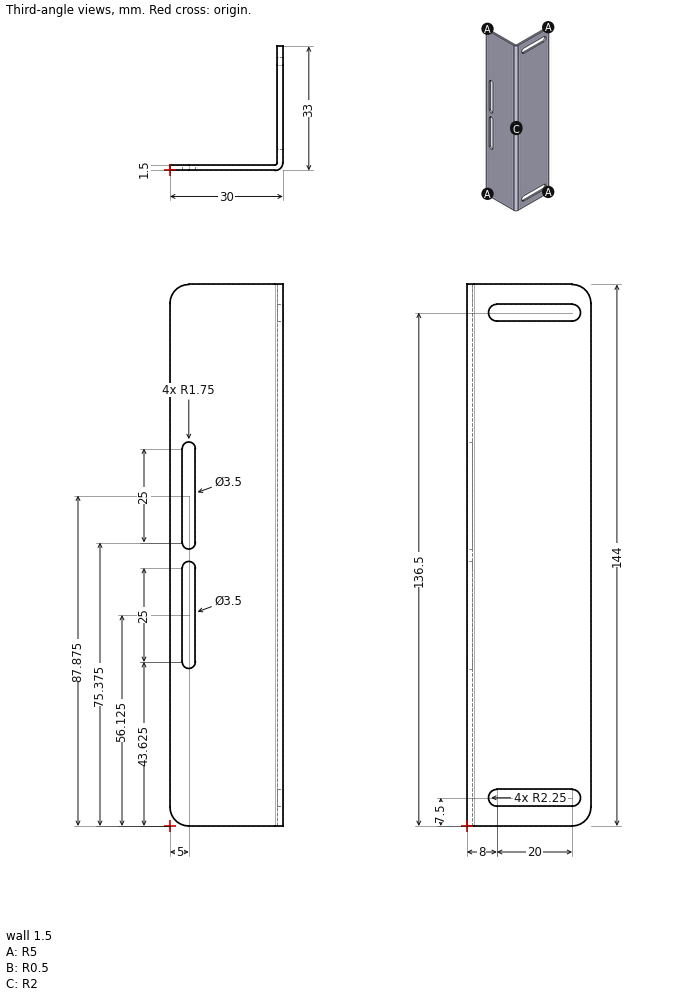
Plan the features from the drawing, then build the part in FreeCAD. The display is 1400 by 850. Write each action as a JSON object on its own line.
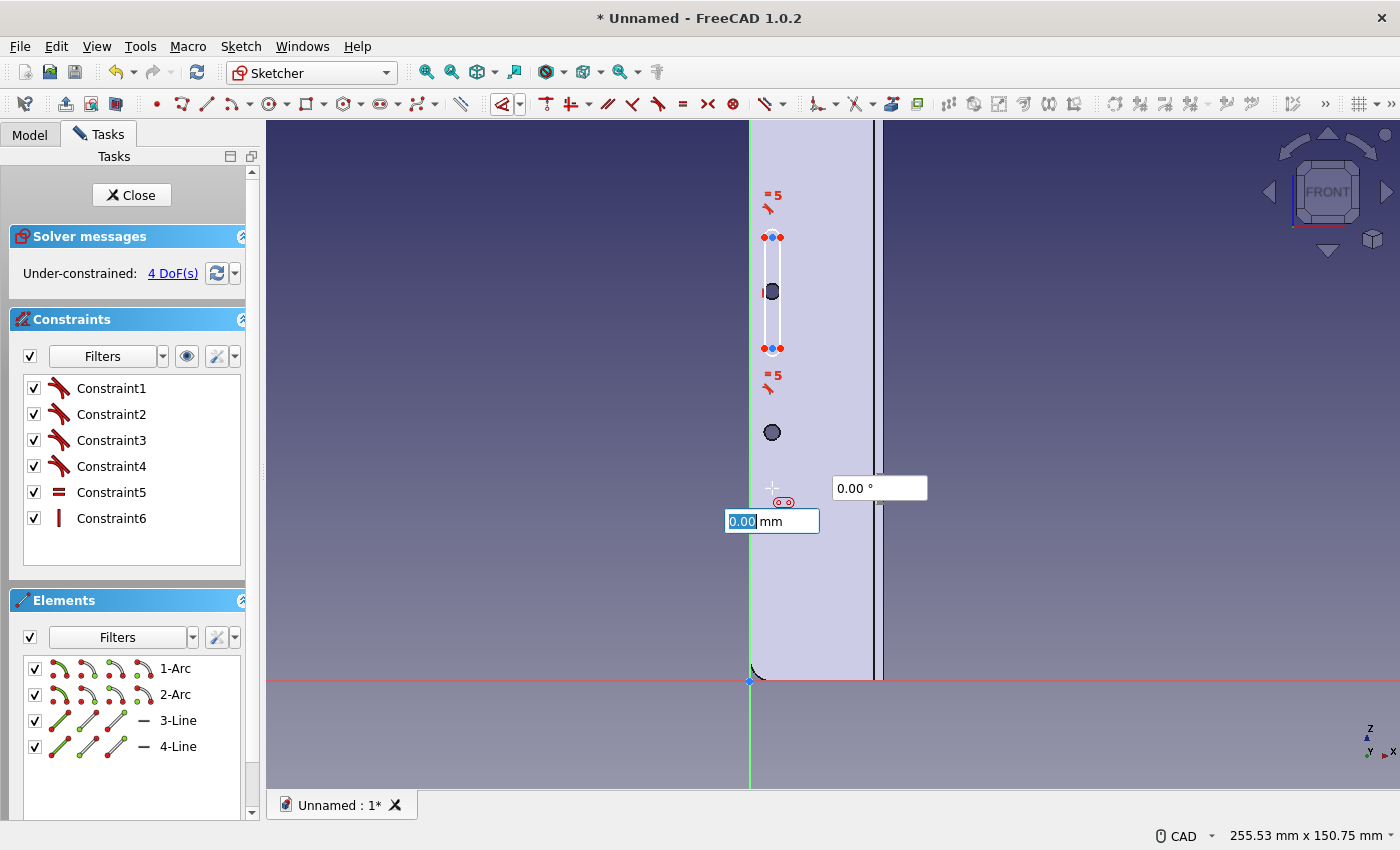
{"action": "left_click", "coordinate": [772, 377]}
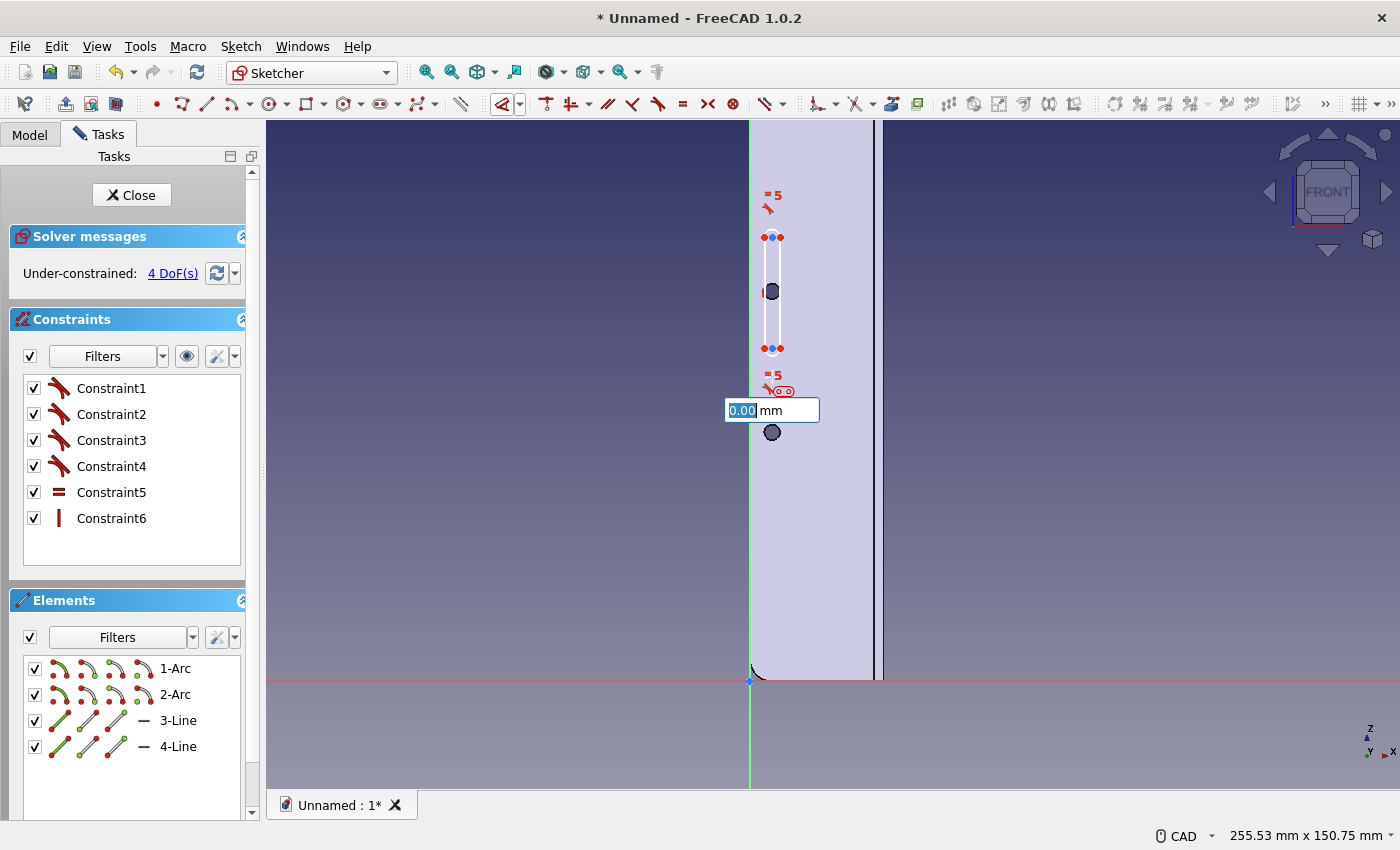
{"action": "scroll", "coordinate": [764, 432], "scroll_direction": "up", "scroll_amount": 4}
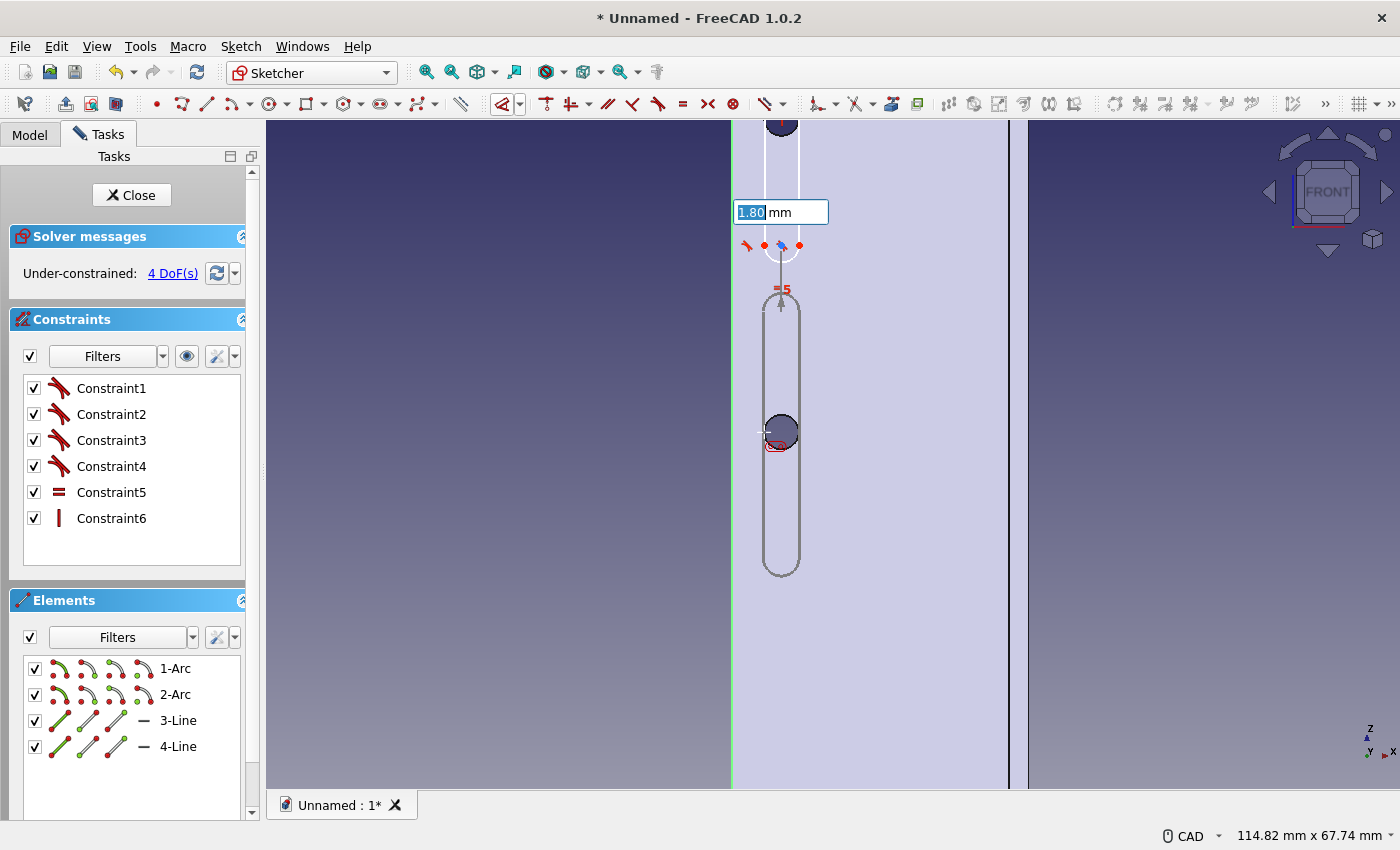
{"action": "left_click", "coordinate": [764, 432]}
{"action": "key", "text": "Escape"}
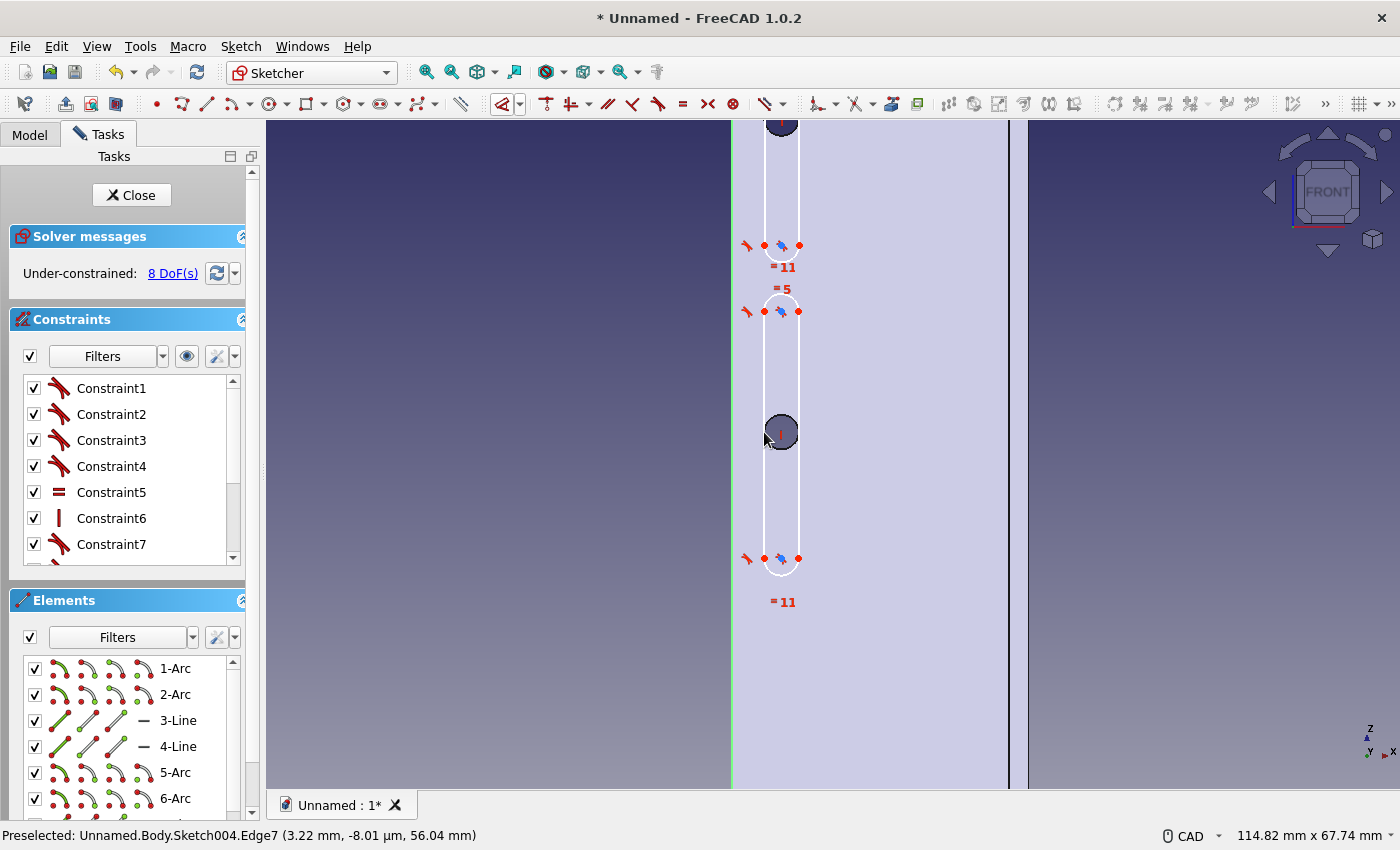
{"action": "left_click", "coordinate": [768, 255]}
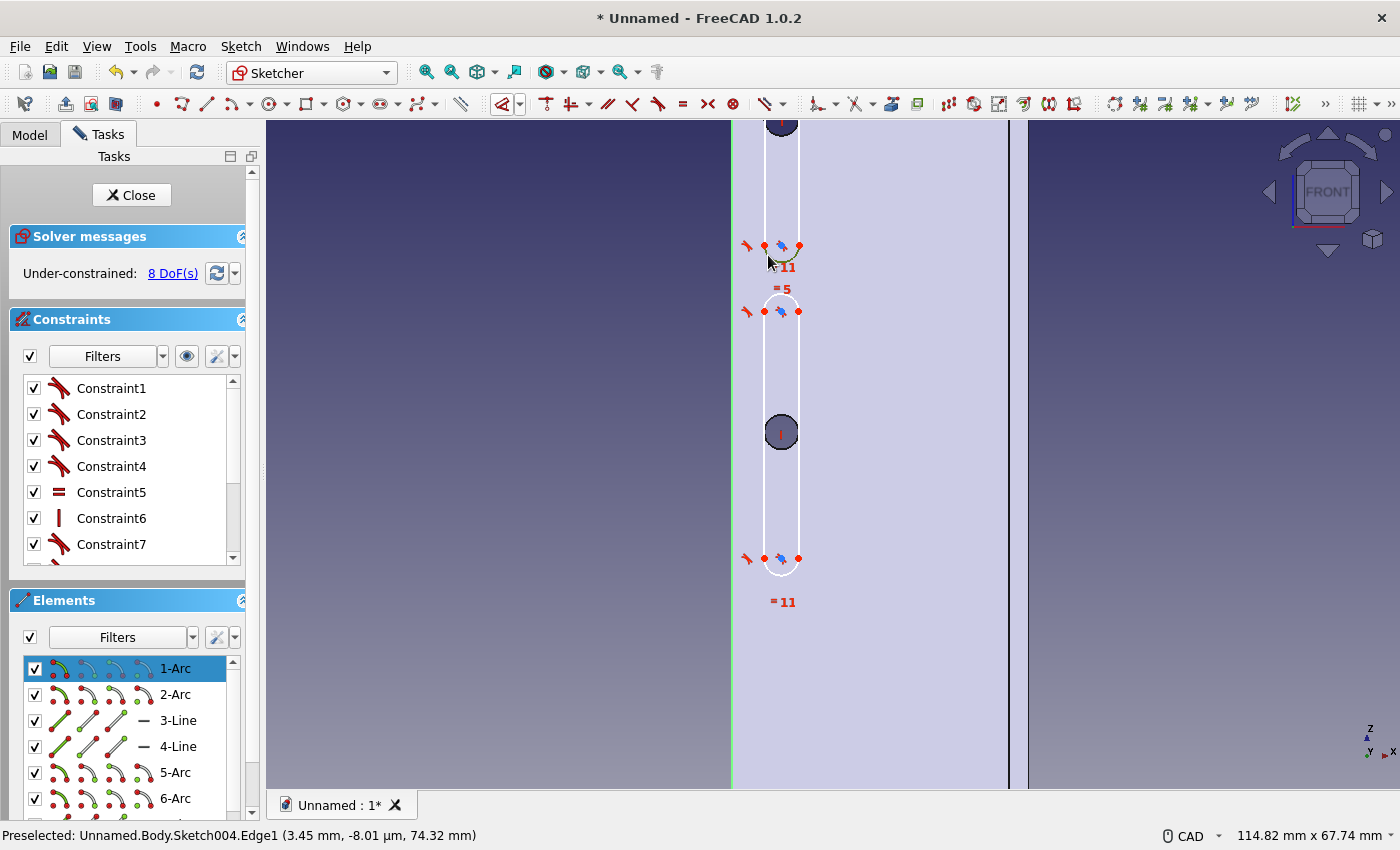
{"action": "left_click", "coordinate": [771, 572]}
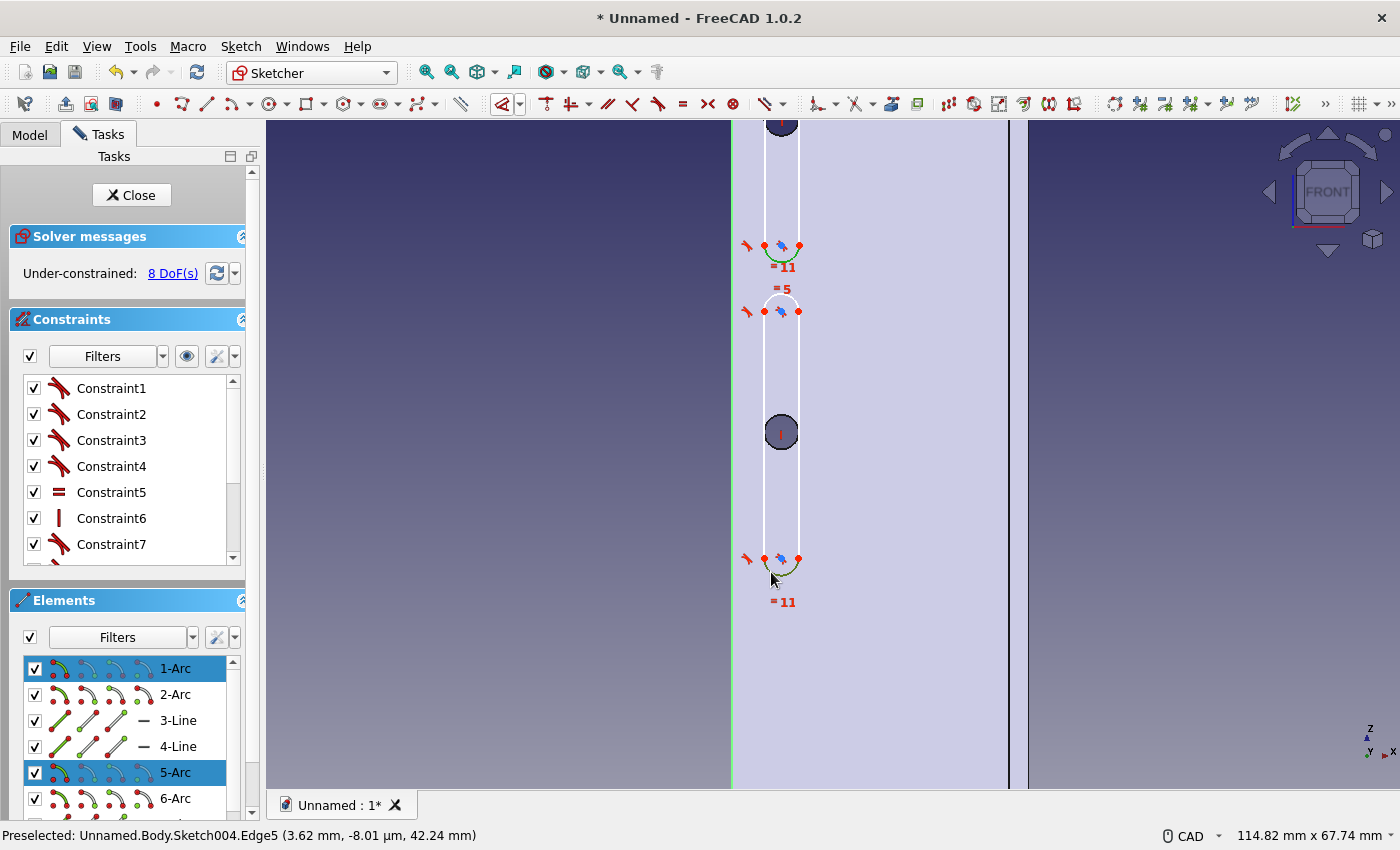
{"action": "left_click", "coordinate": [683, 104]}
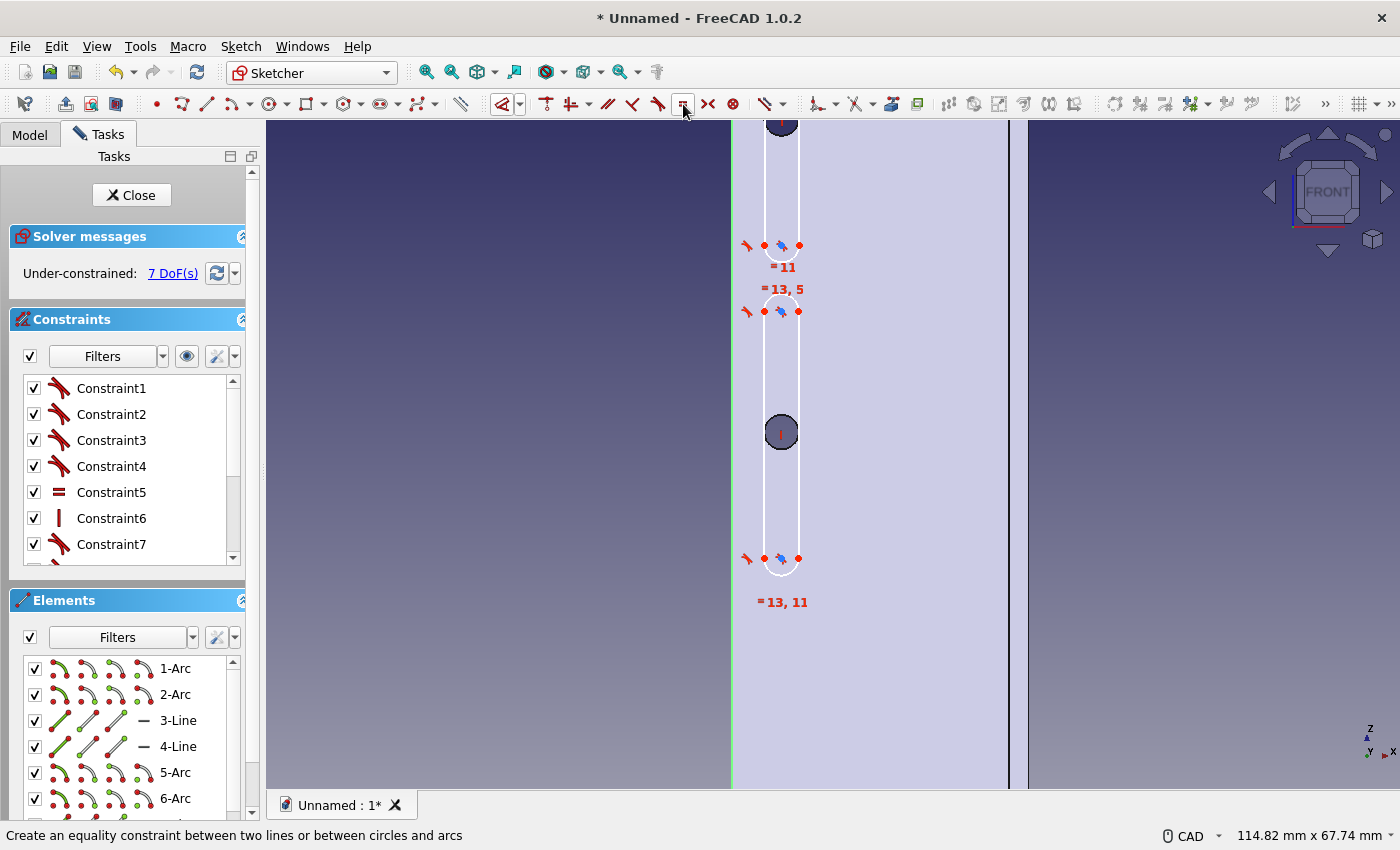
{"action": "scroll", "coordinate": [772, 259], "scroll_direction": "up", "scroll_amount": 5}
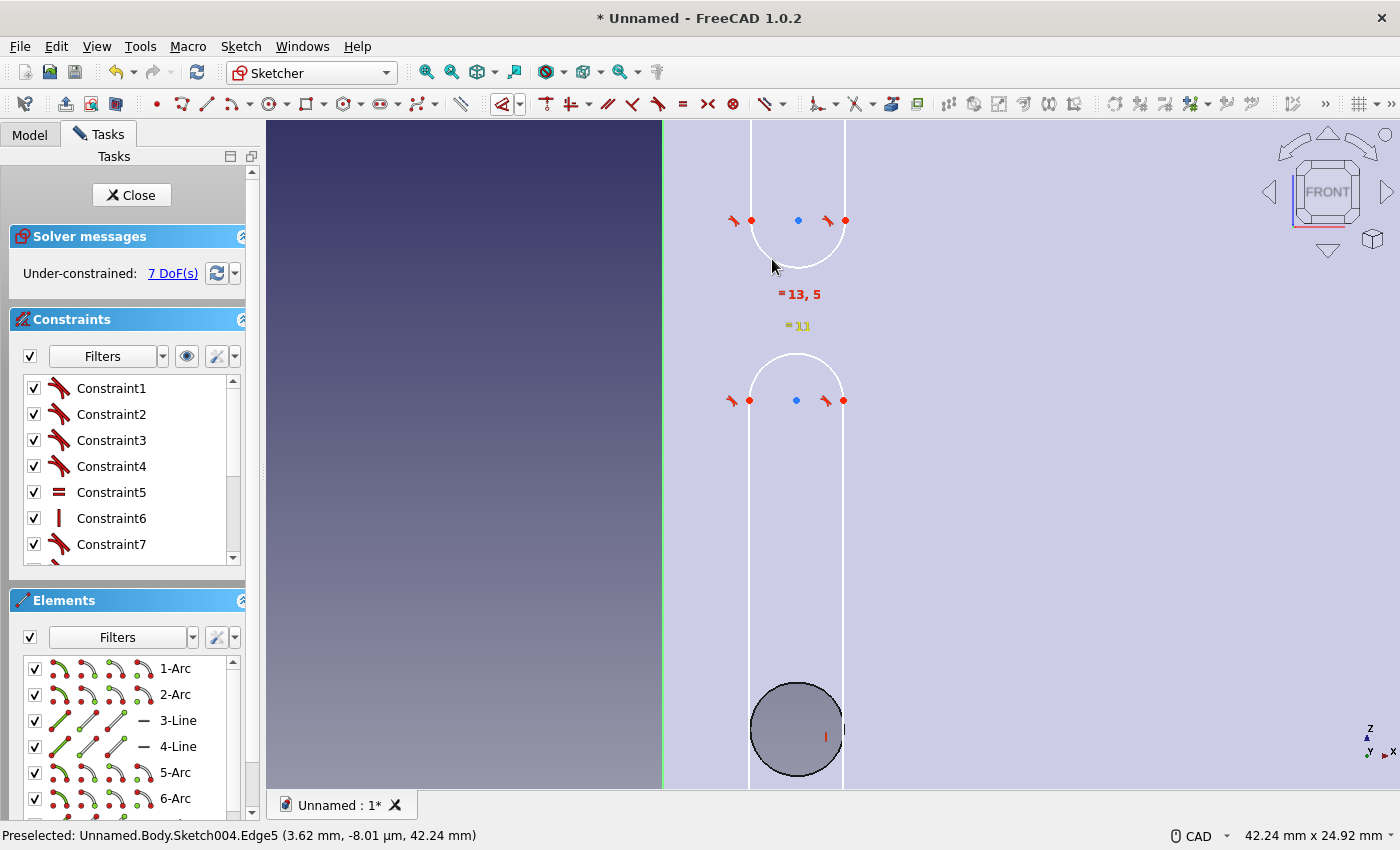
{"action": "left_click", "coordinate": [771, 259]}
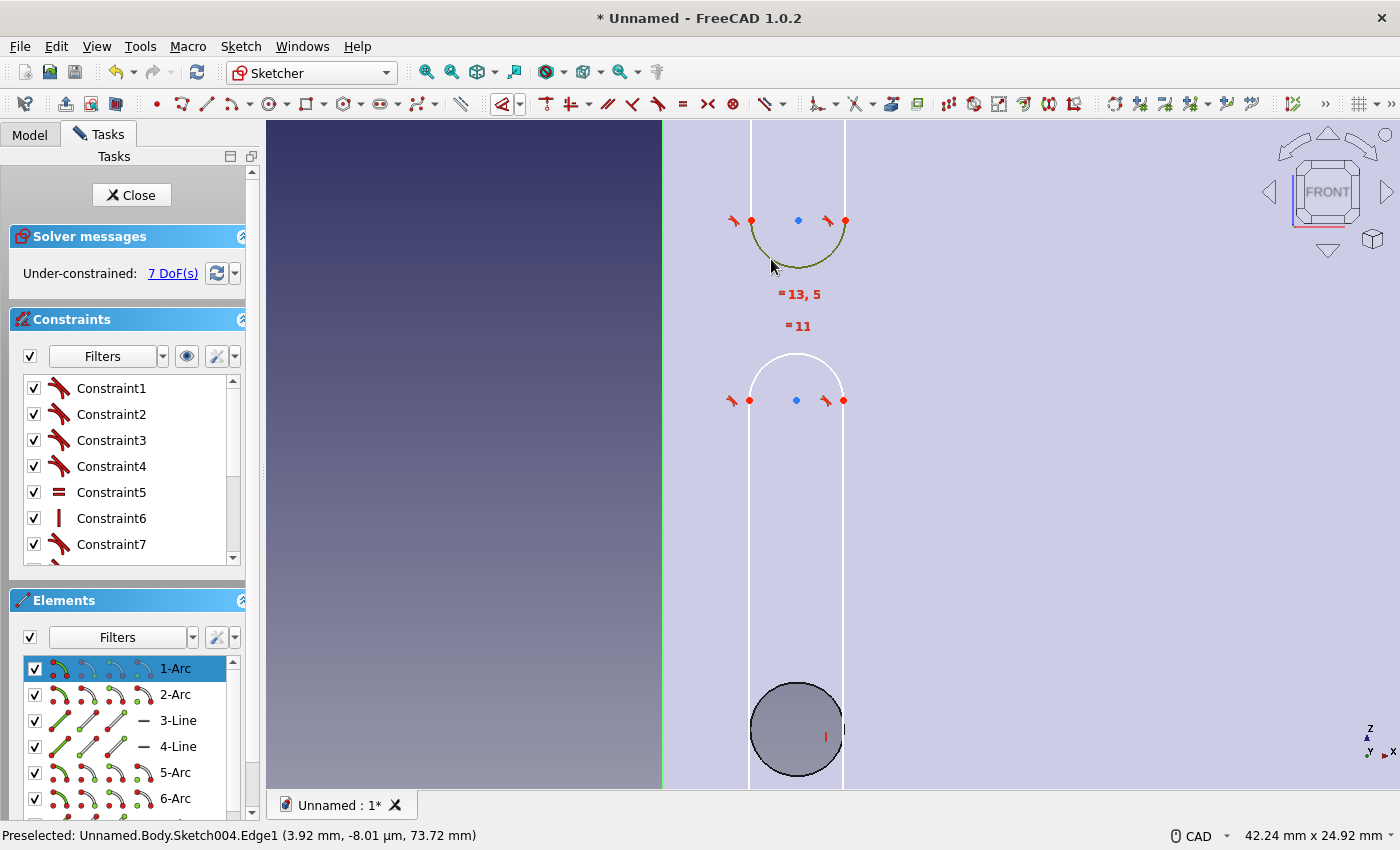
{"action": "key", "text": "k r"}